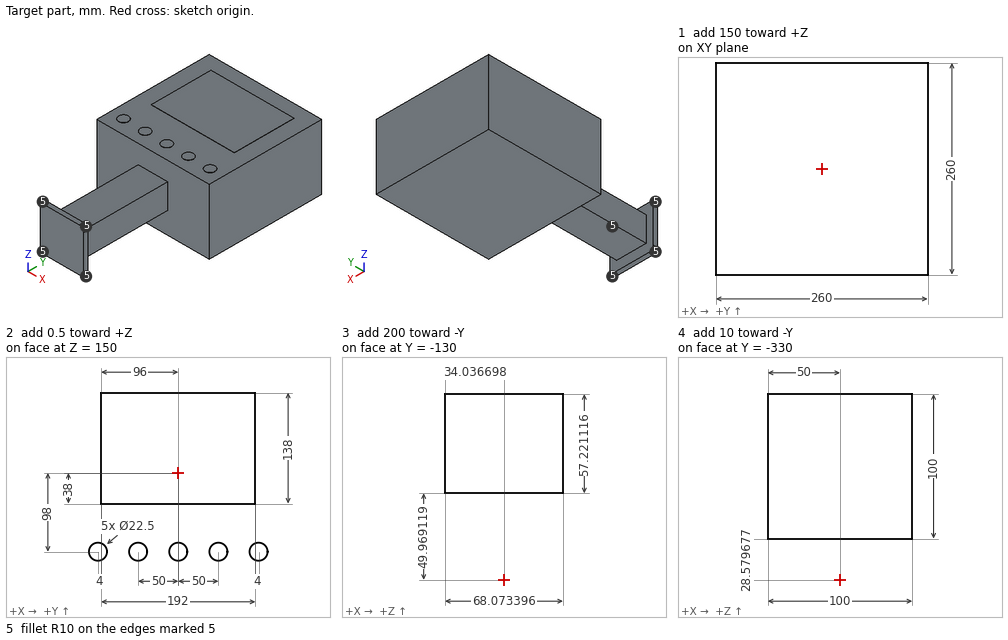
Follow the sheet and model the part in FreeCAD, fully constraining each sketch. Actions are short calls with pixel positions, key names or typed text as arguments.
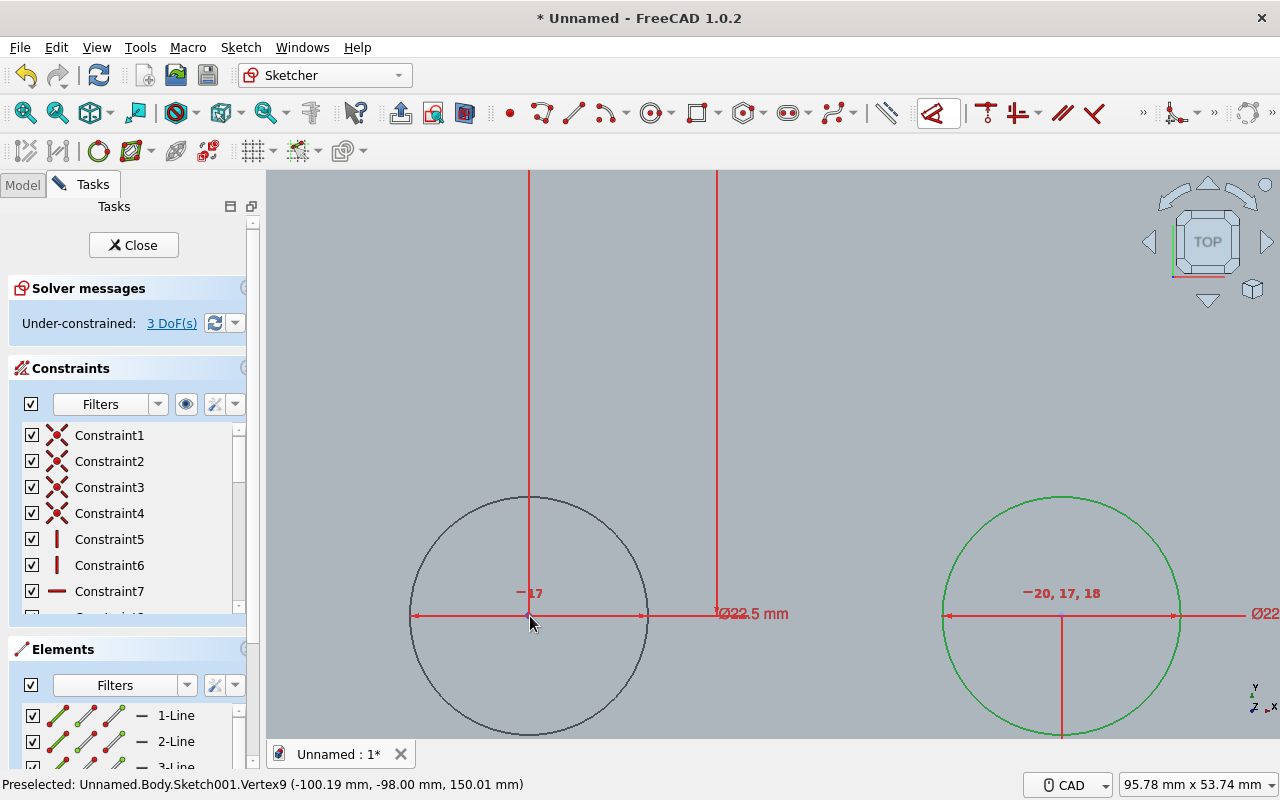
scroll(529, 618, down, 9)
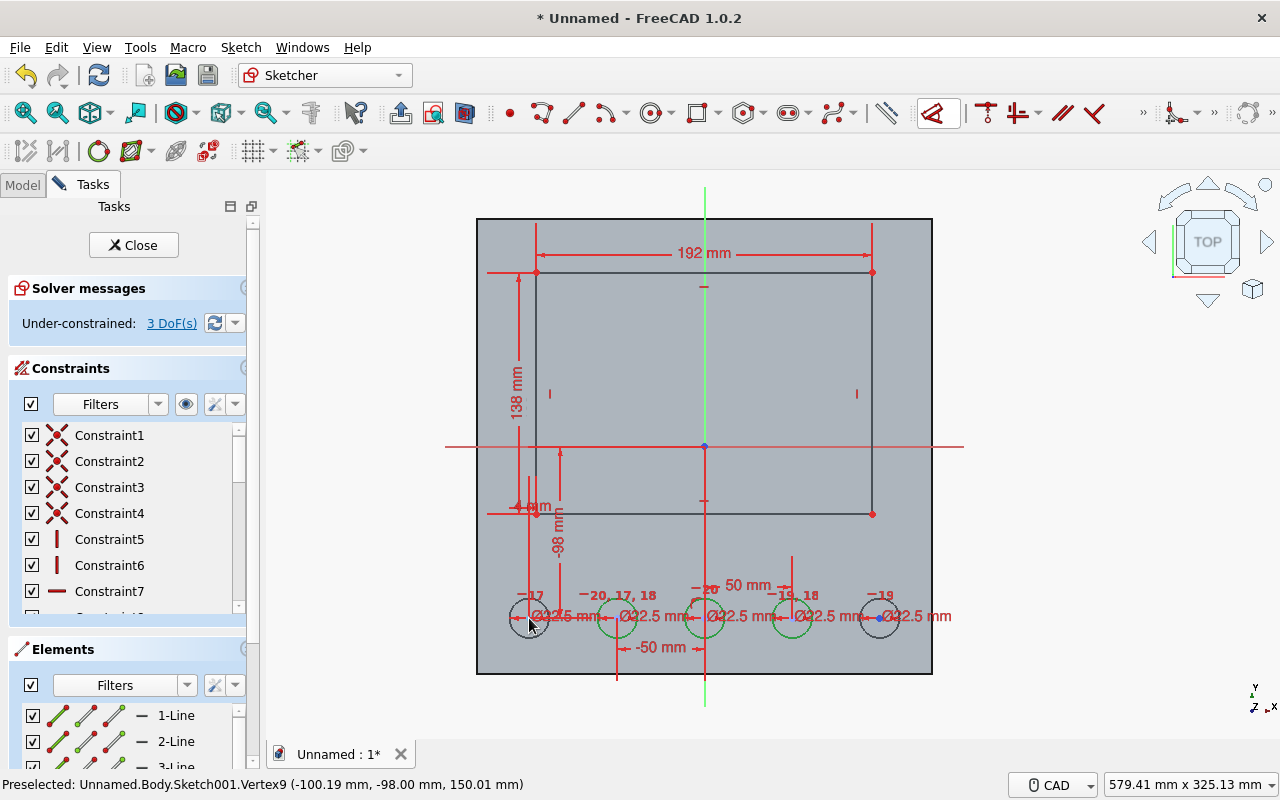
scroll(872, 514, up, 9)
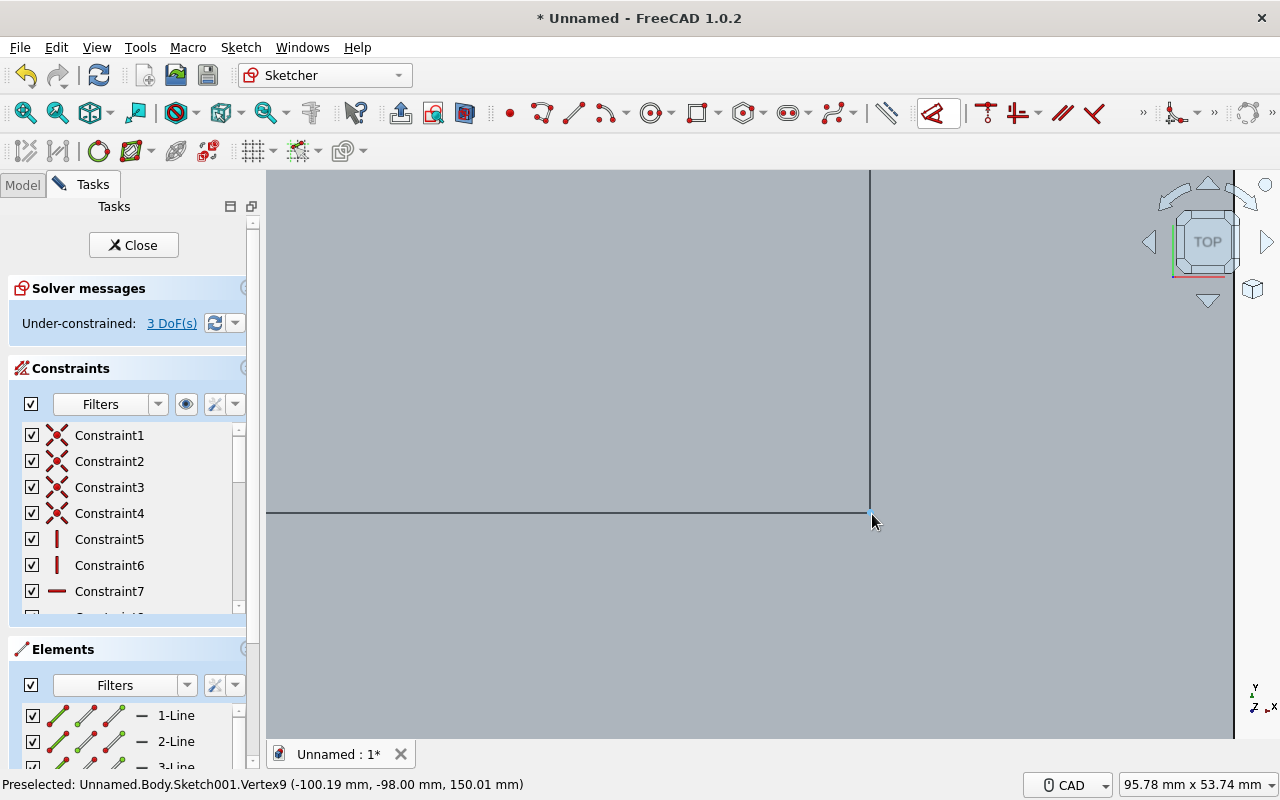
click(870, 513)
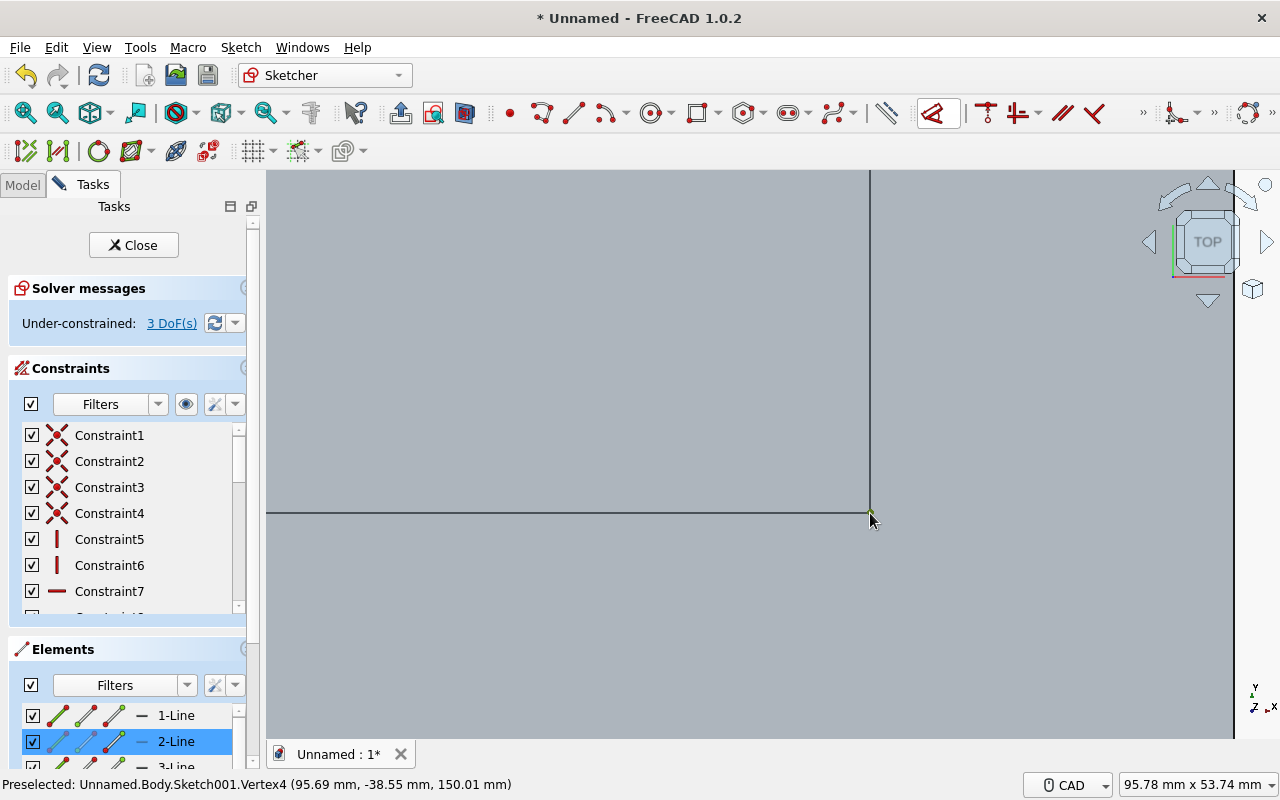
scroll(872, 514, down, 9)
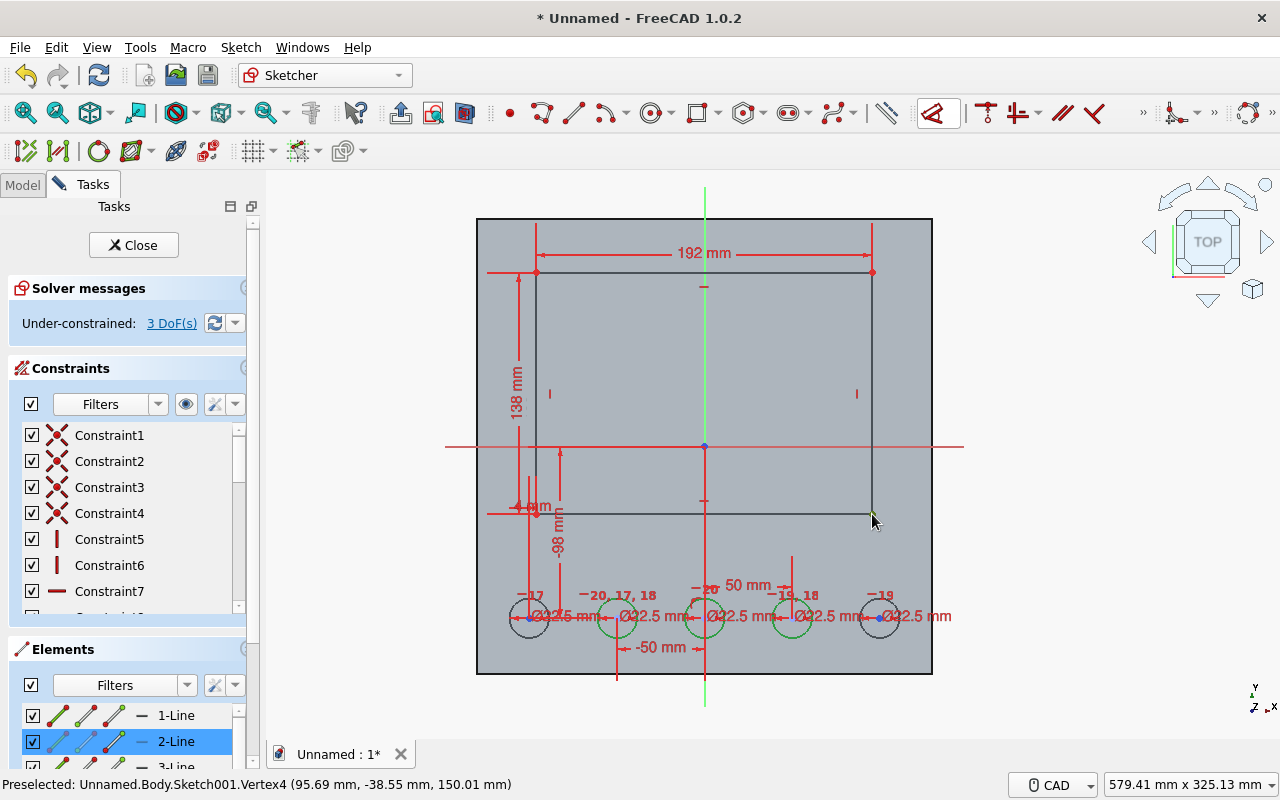
scroll(880, 618, up, 9)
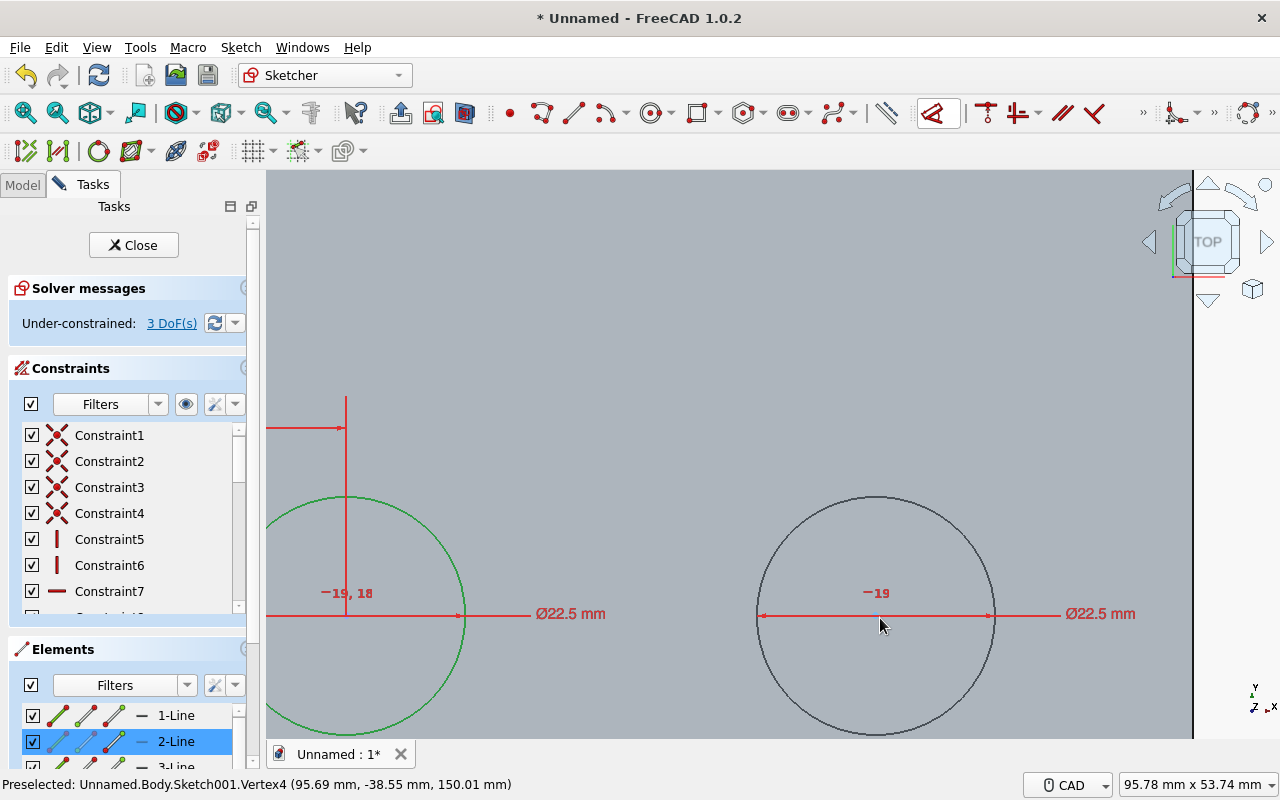
click(876, 616)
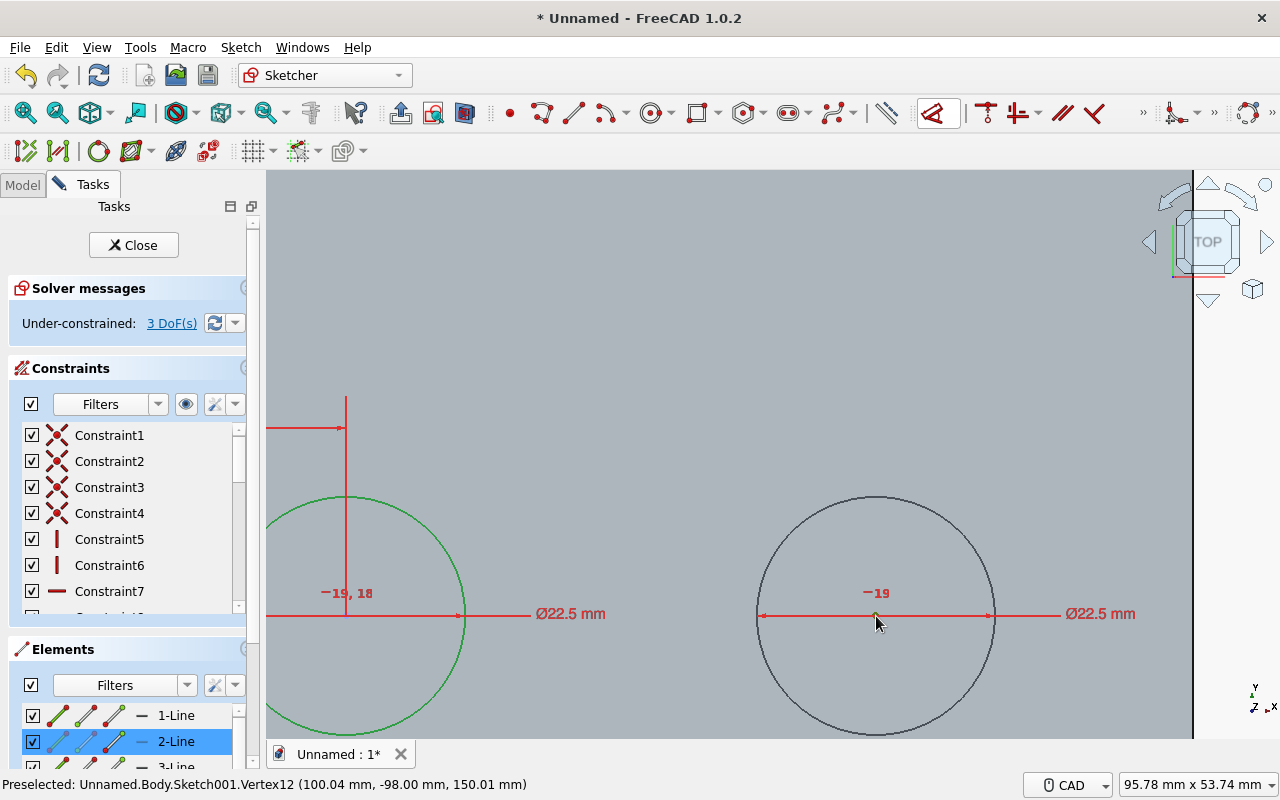
click(954, 114)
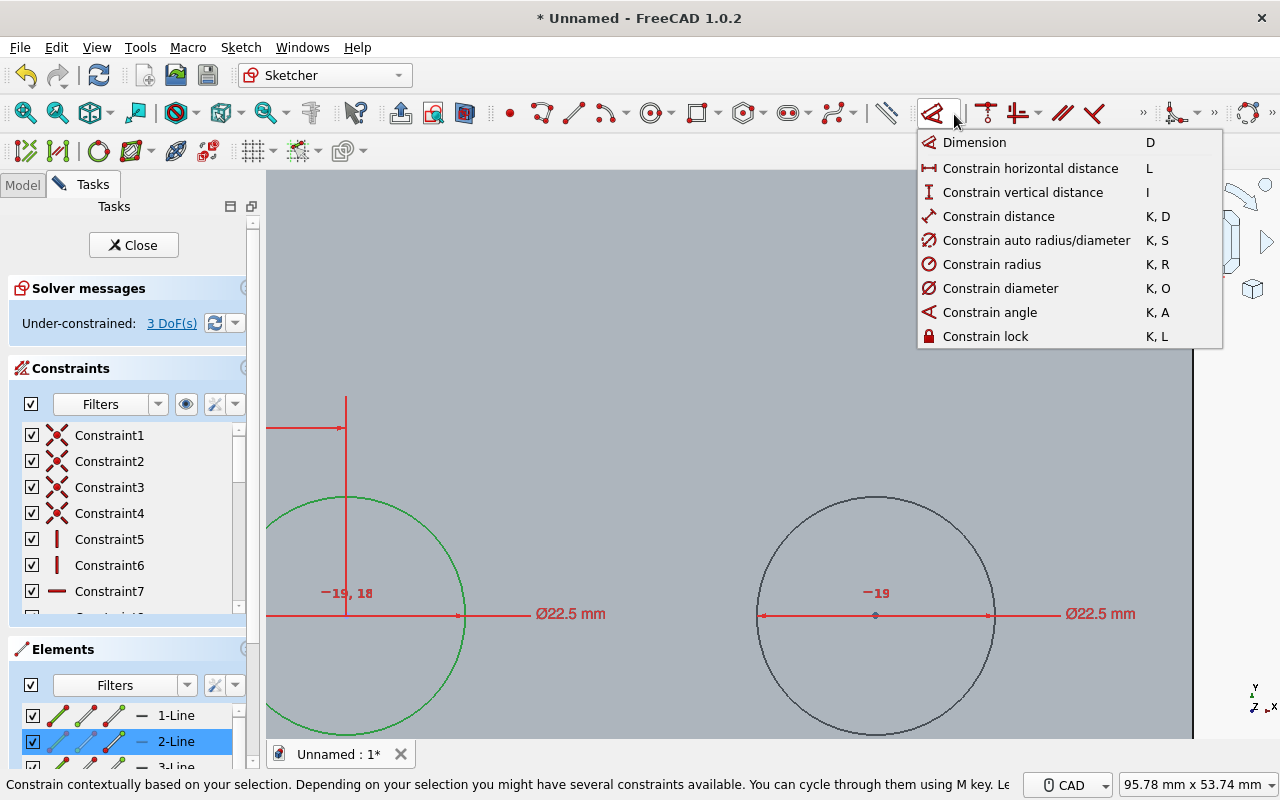
click(1070, 168)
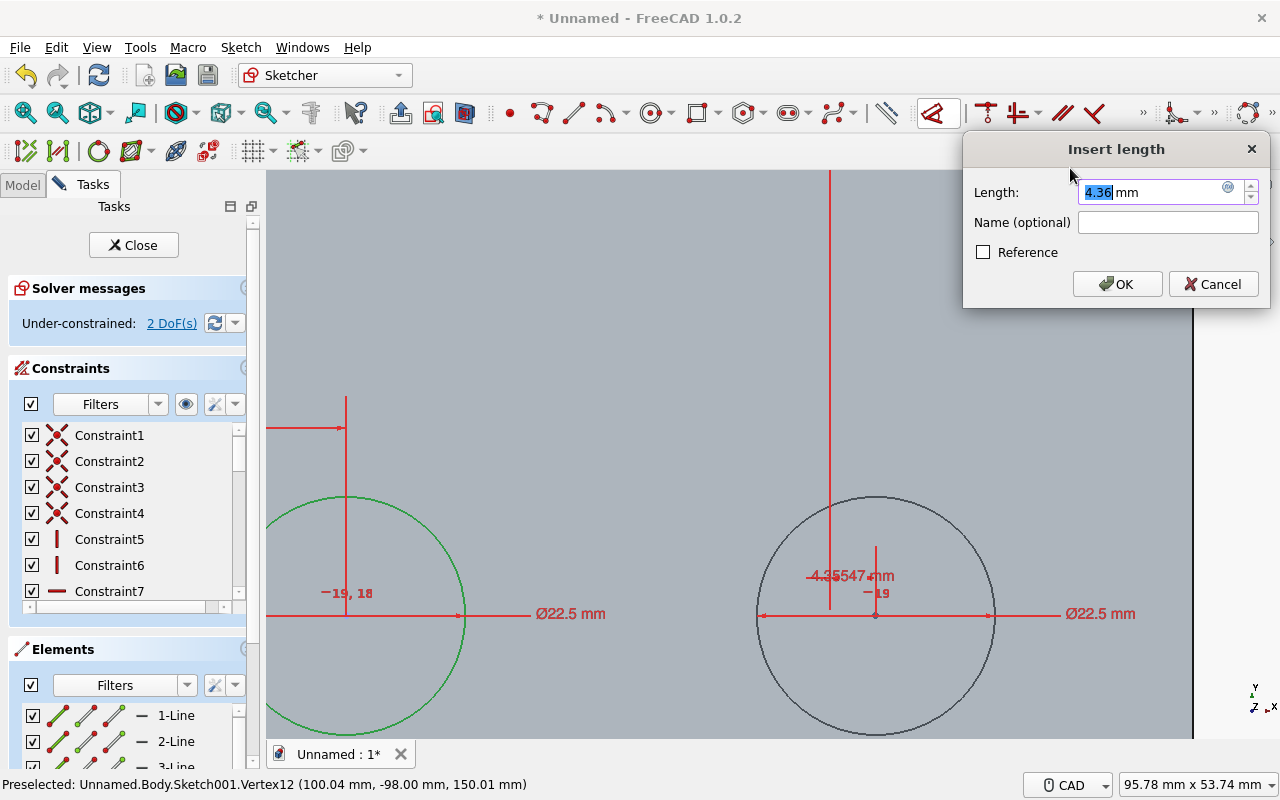
text(4)
key(Return)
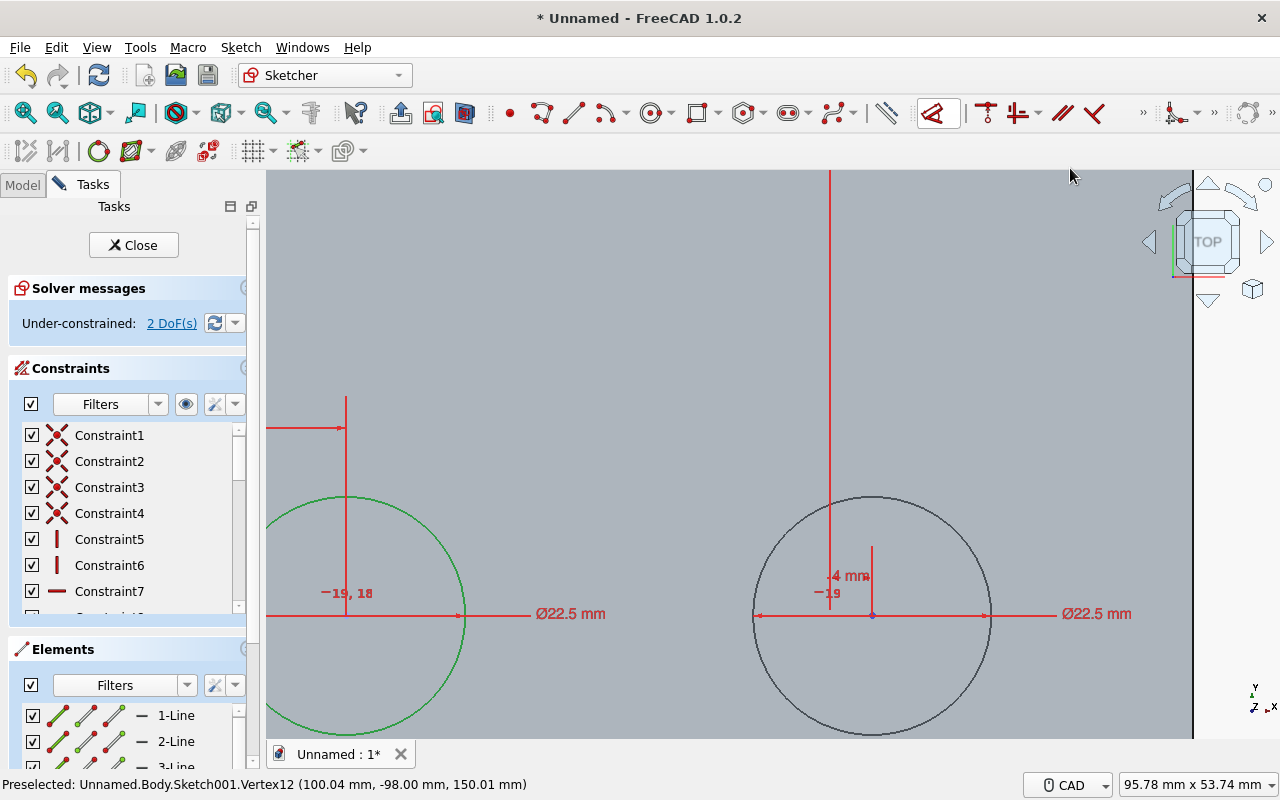
scroll(880, 618, down, 9)